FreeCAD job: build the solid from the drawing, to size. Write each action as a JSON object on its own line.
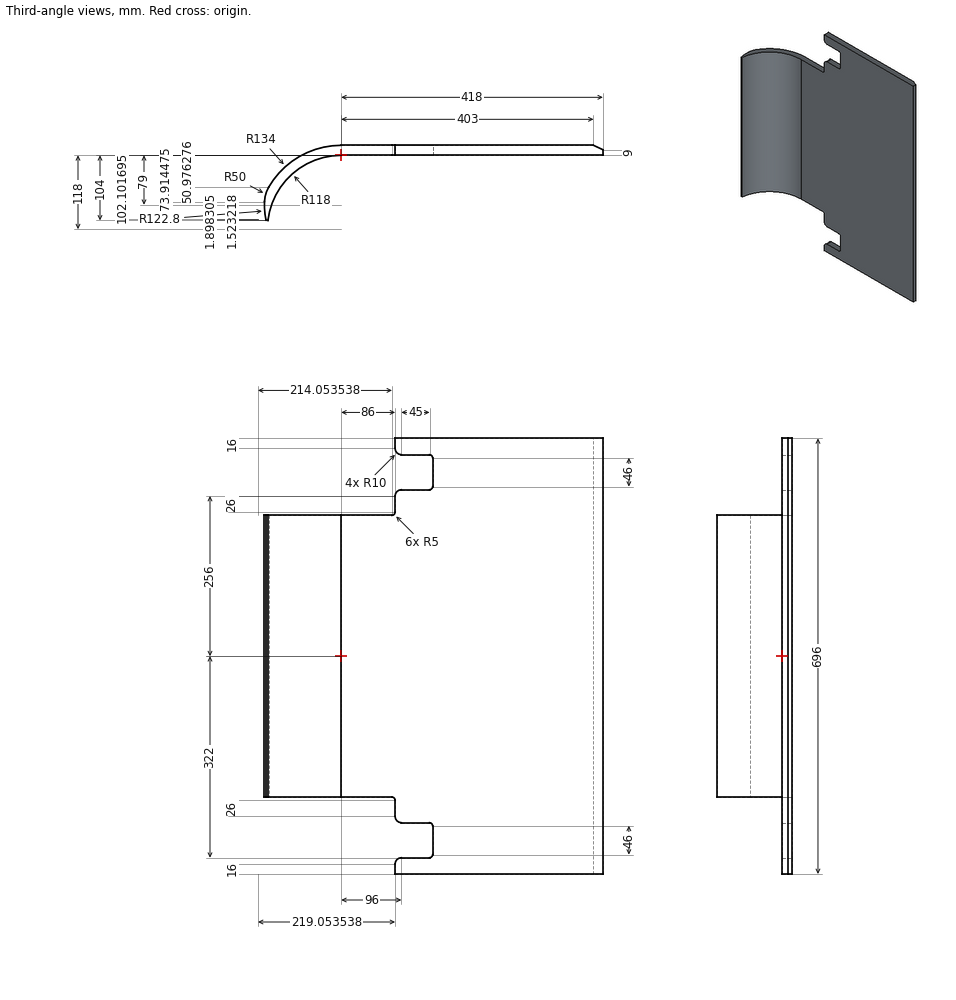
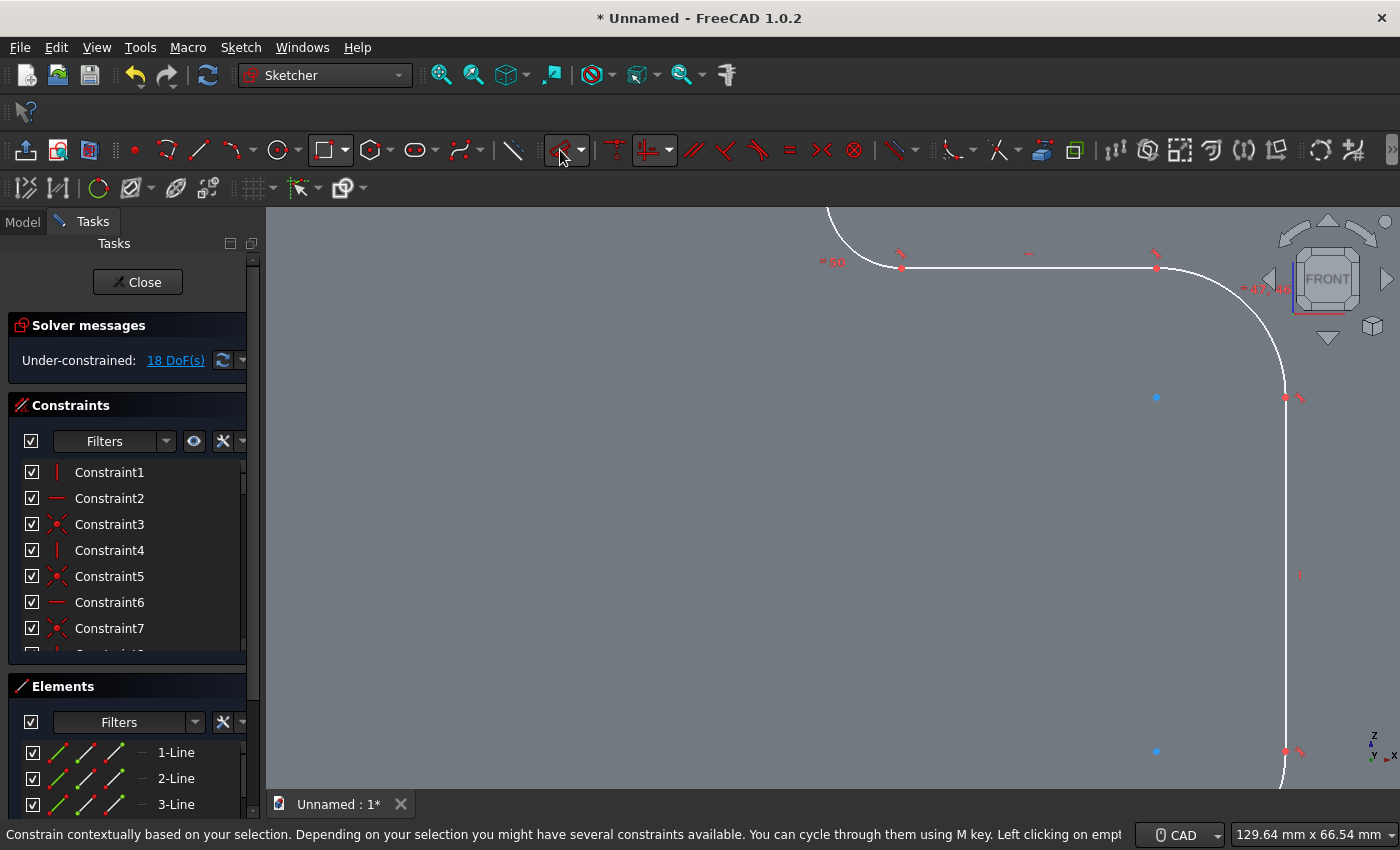
{"action": "scroll", "coordinate": [811, 660], "scroll_direction": "down", "scroll_amount": 14}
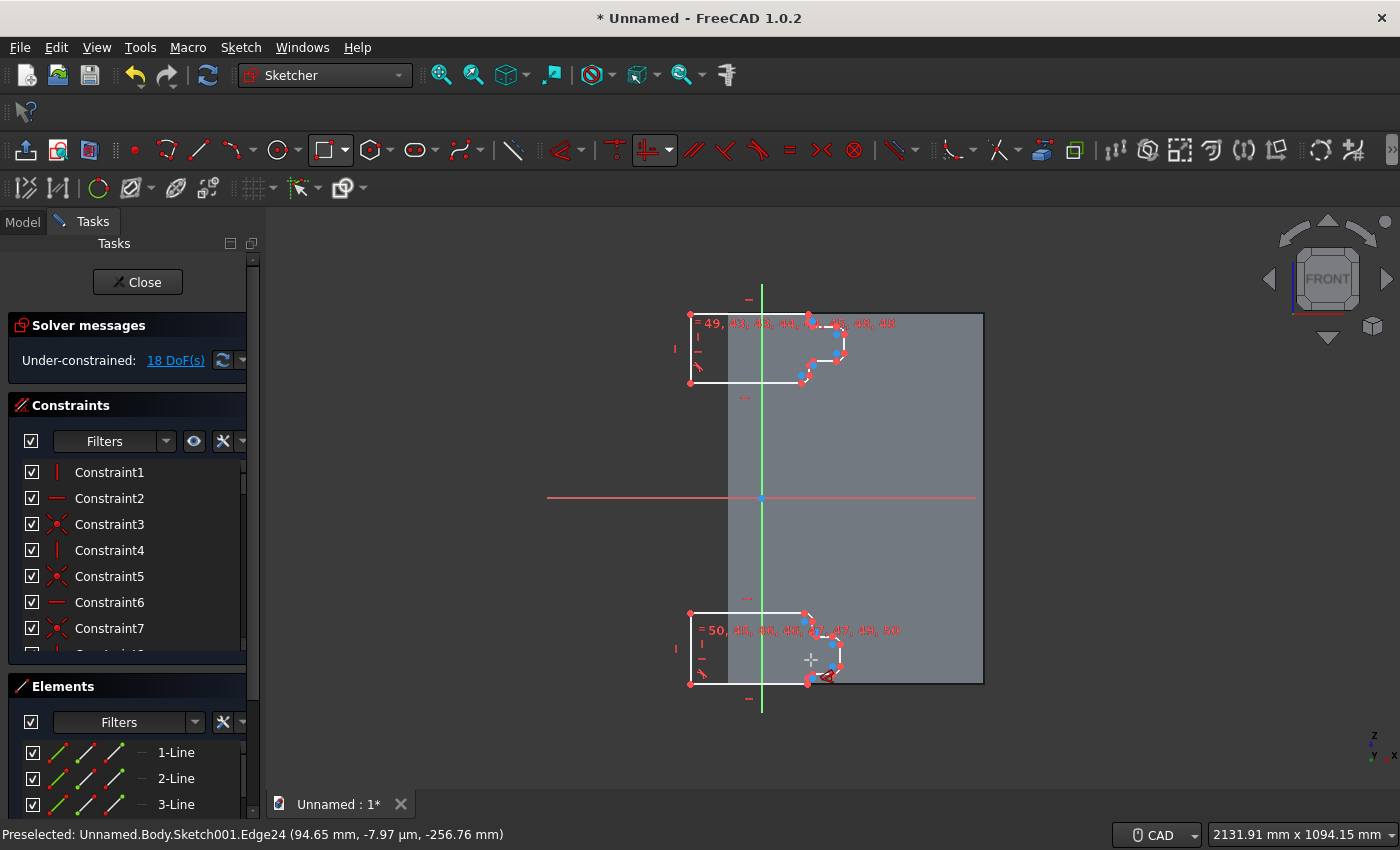
{"action": "scroll", "coordinate": [805, 382], "scroll_direction": "up", "scroll_amount": 14}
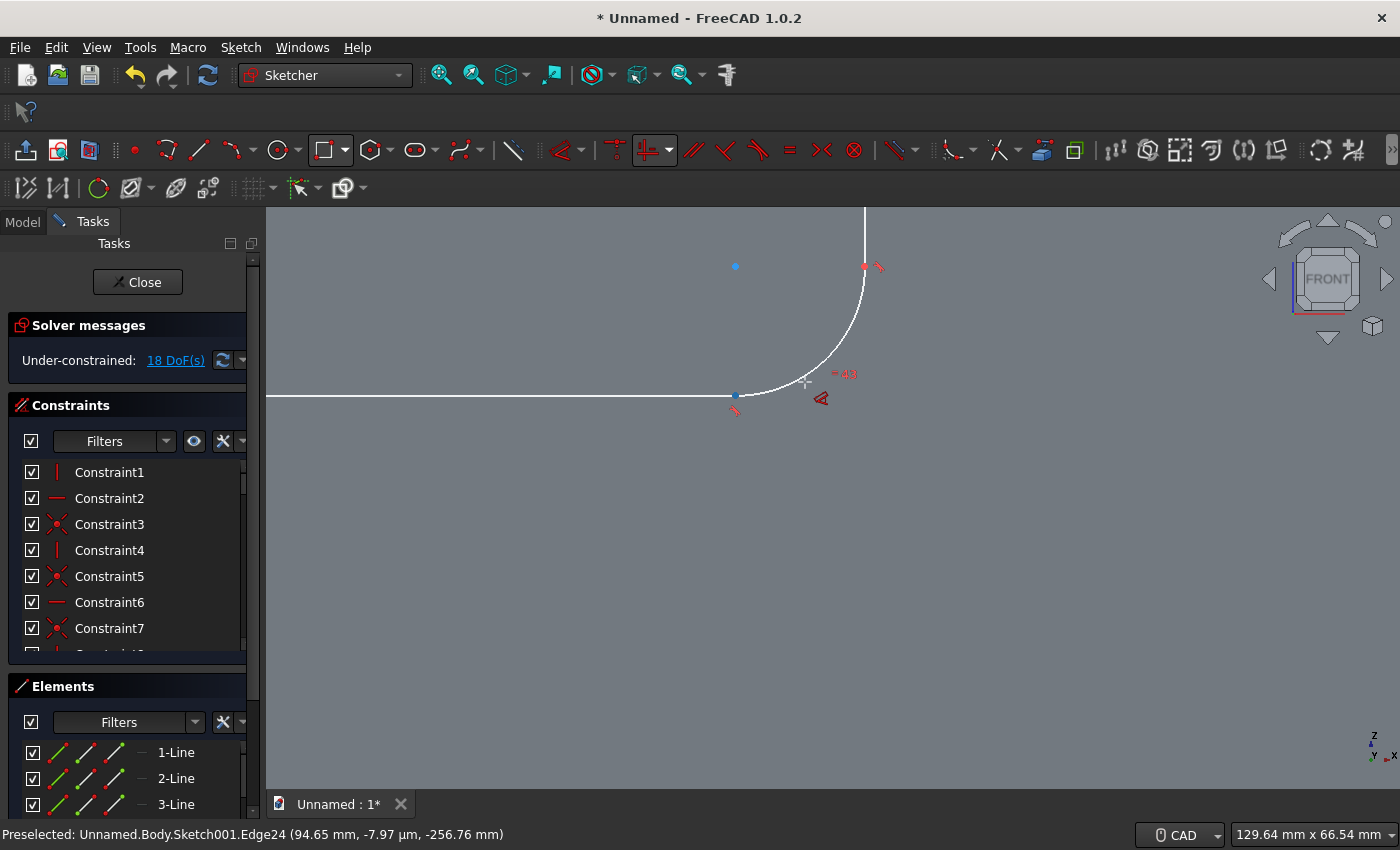
{"action": "left_click", "coordinate": [794, 382]}
{"action": "left_click", "coordinate": [808, 411]}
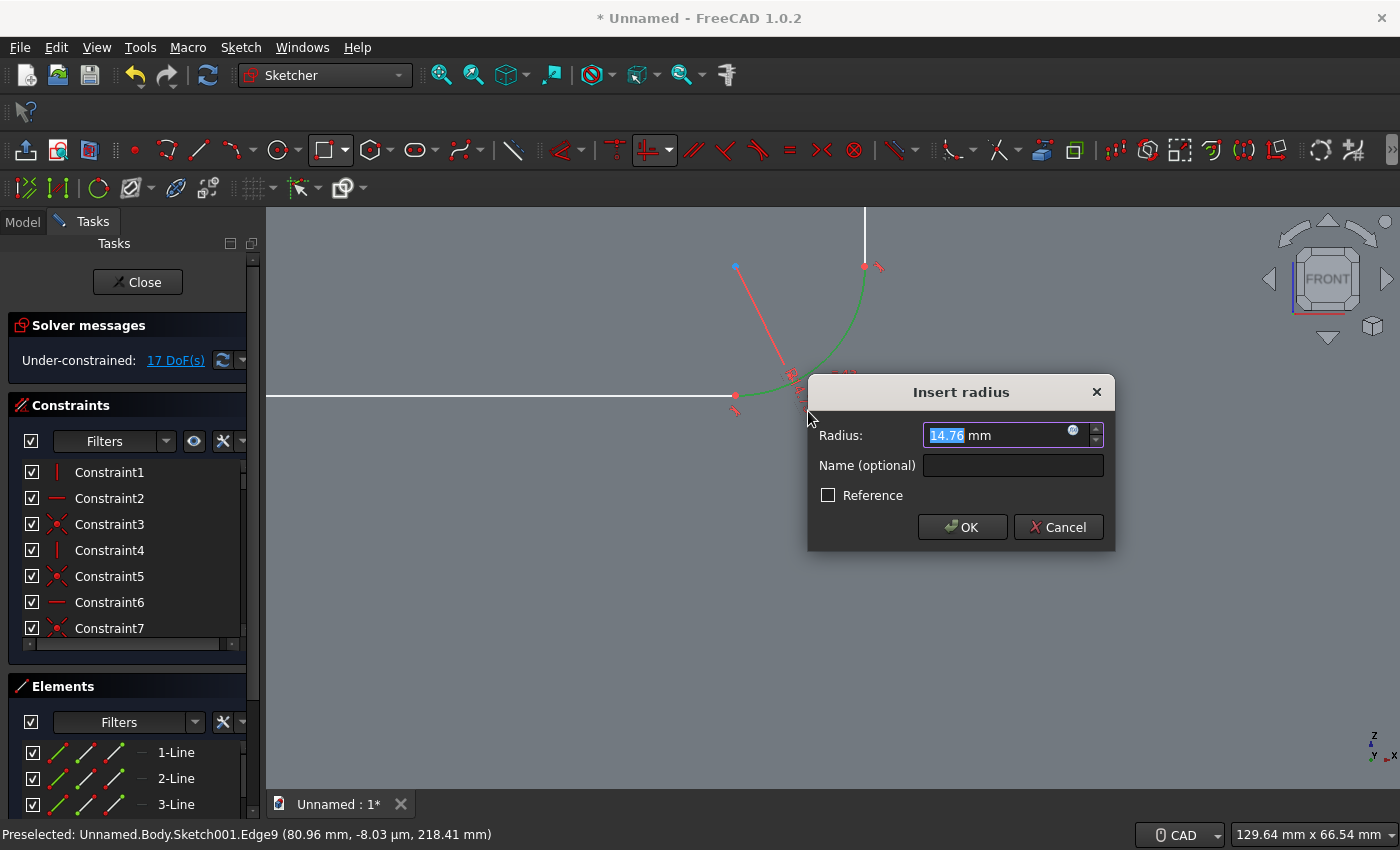
{"action": "type", "text": "5"}
{"action": "key", "text": "Return"}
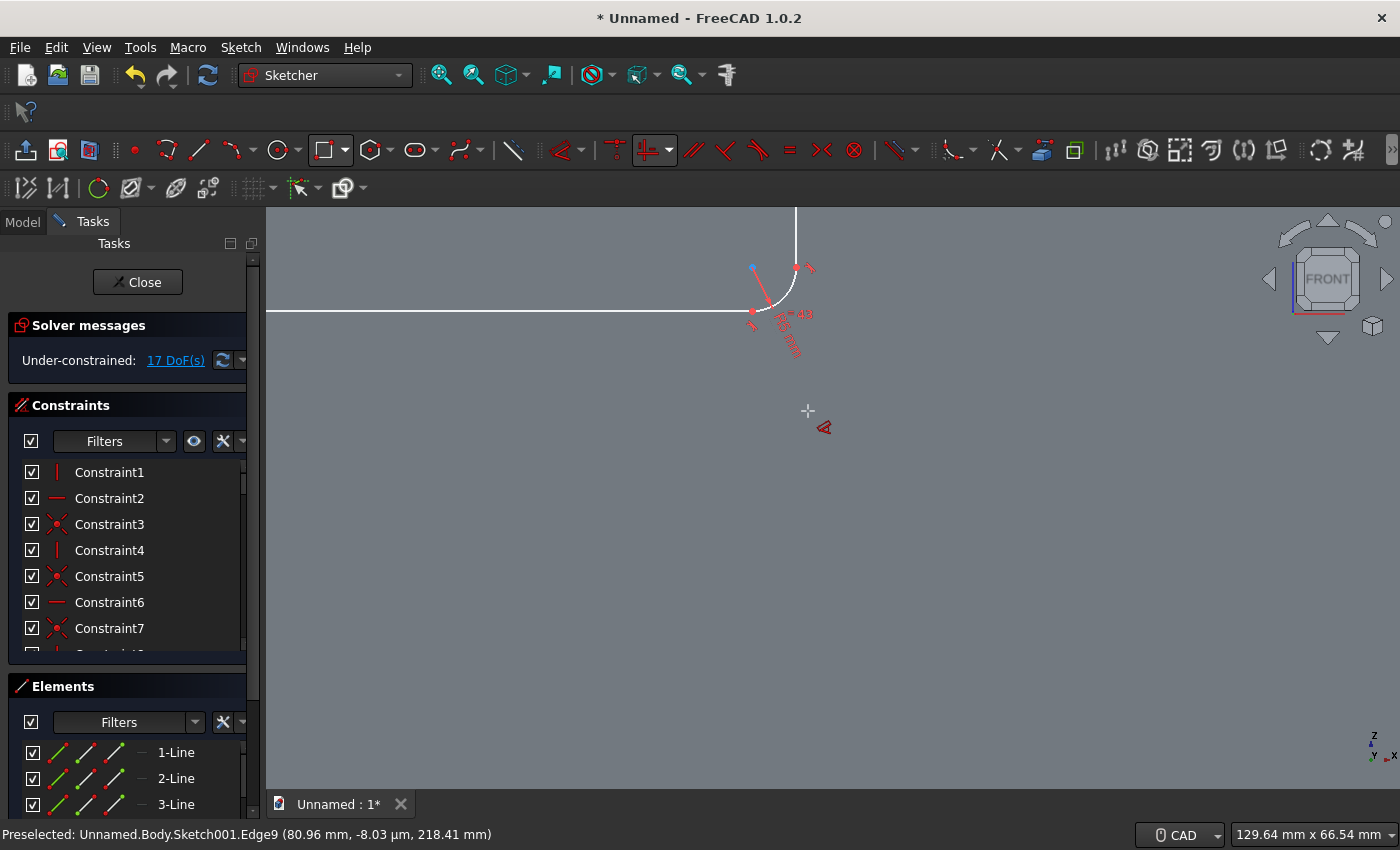
{"action": "scroll", "coordinate": [805, 382], "scroll_direction": "down", "scroll_amount": 14}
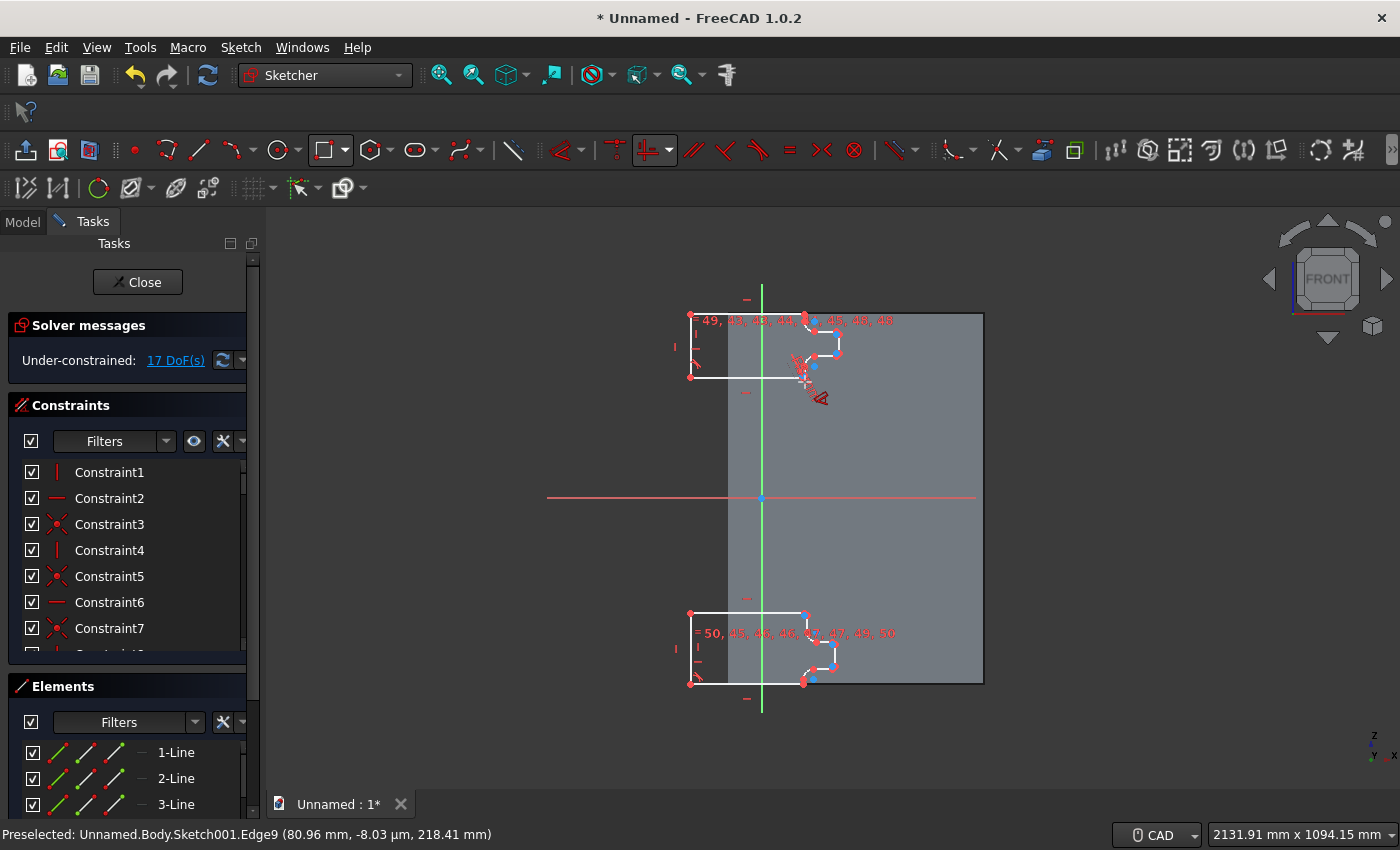
{"action": "scroll", "coordinate": [806, 326], "scroll_direction": "up", "scroll_amount": 11}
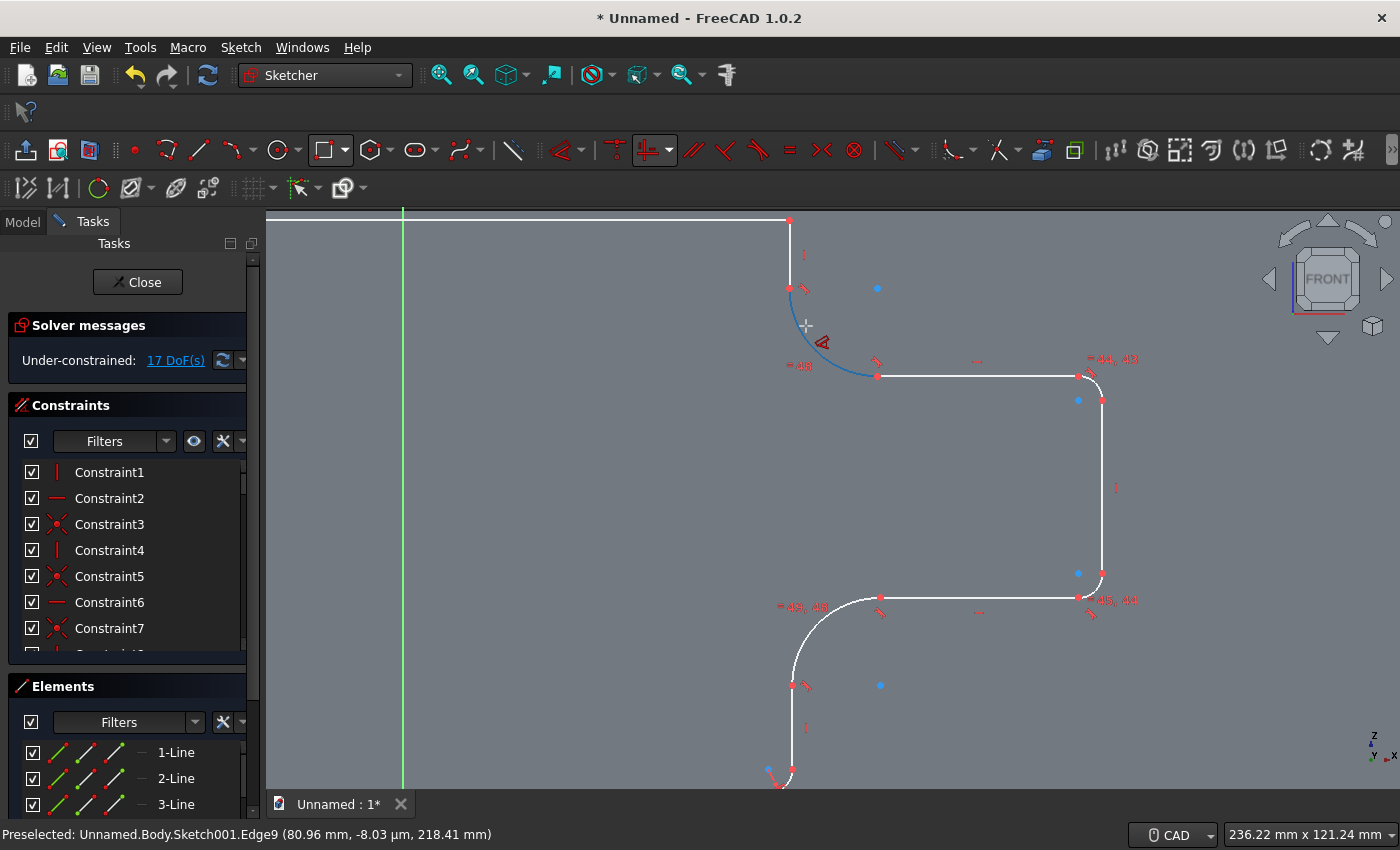
{"action": "left_click", "coordinate": [799, 328]}
{"action": "left_click", "coordinate": [770, 342]}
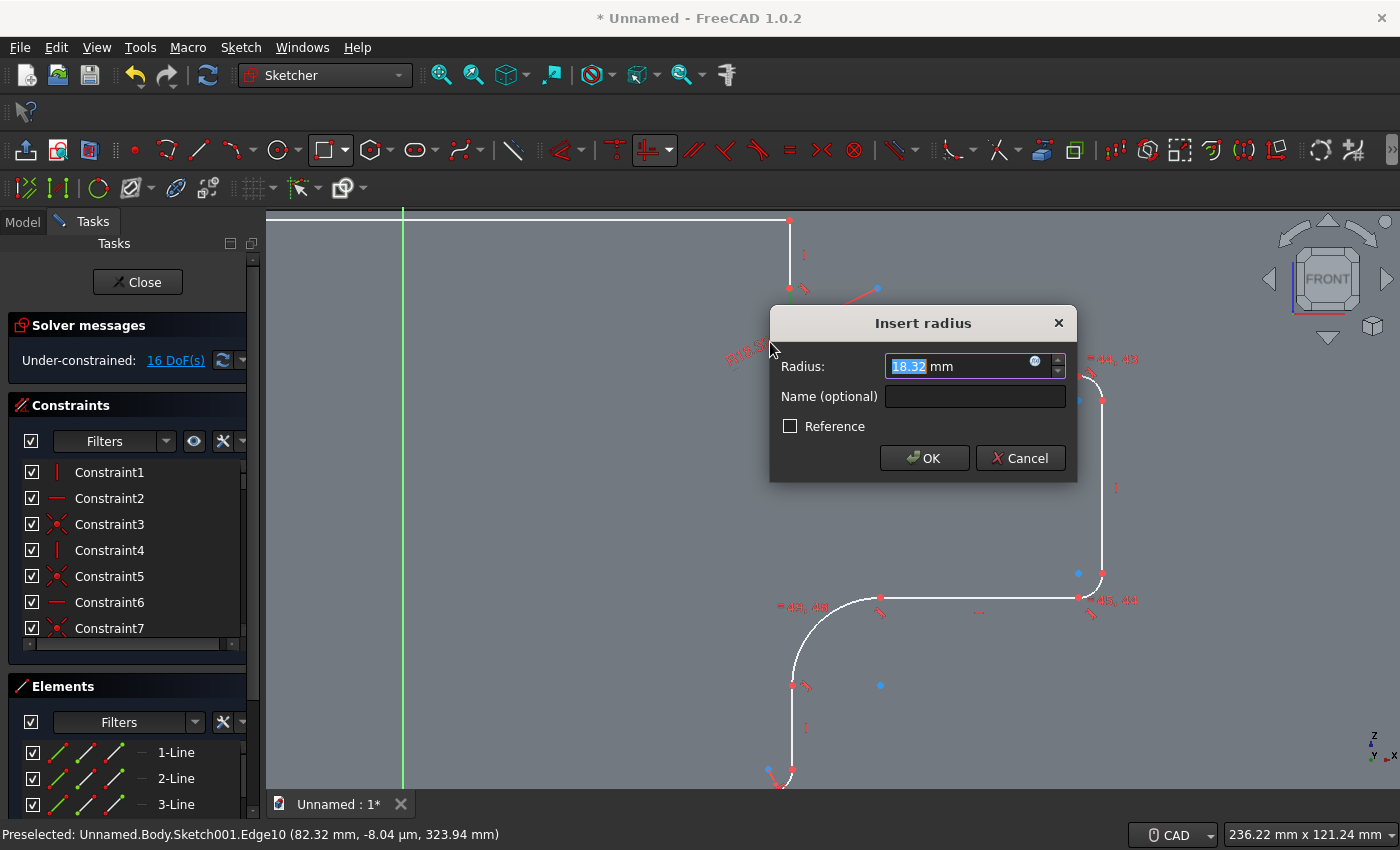
{"action": "type", "text": "10"}
{"action": "key", "text": "Return"}